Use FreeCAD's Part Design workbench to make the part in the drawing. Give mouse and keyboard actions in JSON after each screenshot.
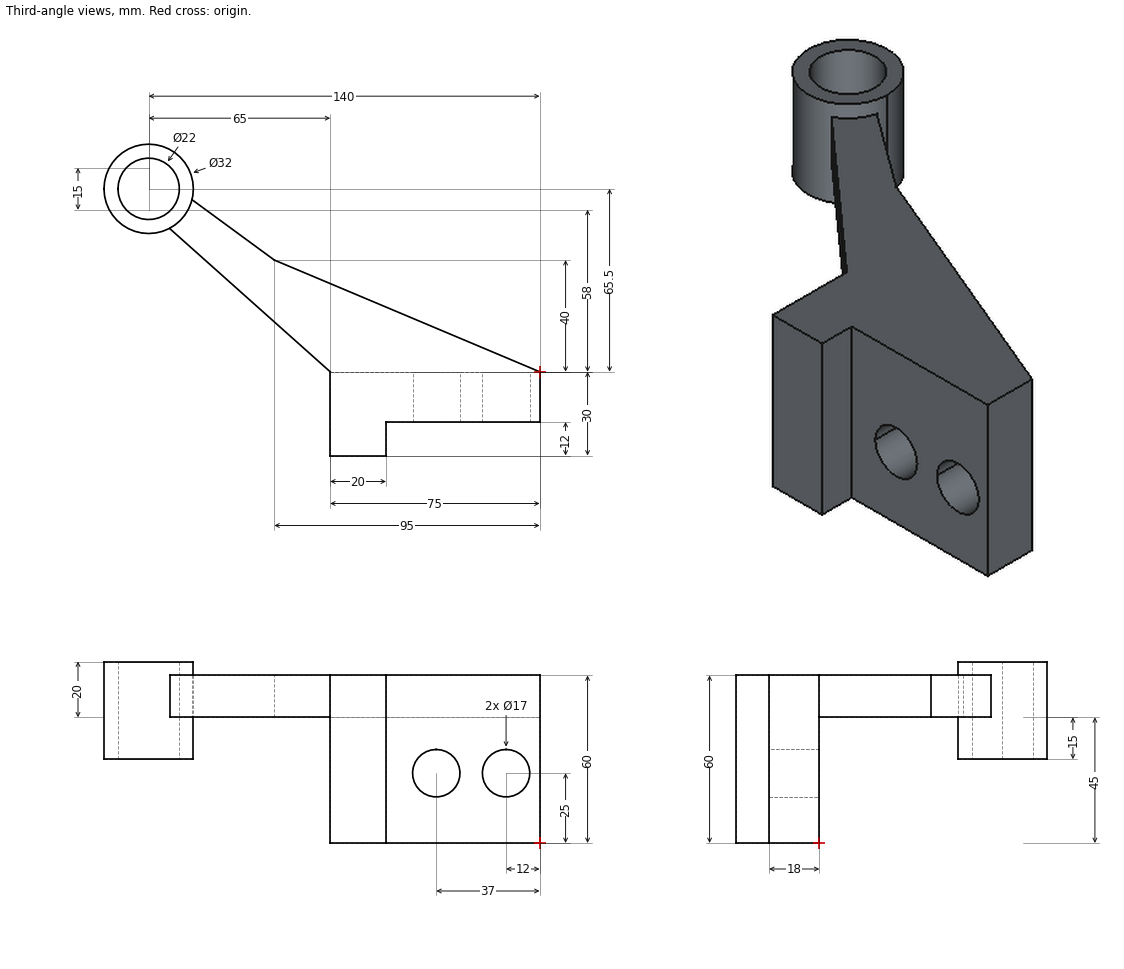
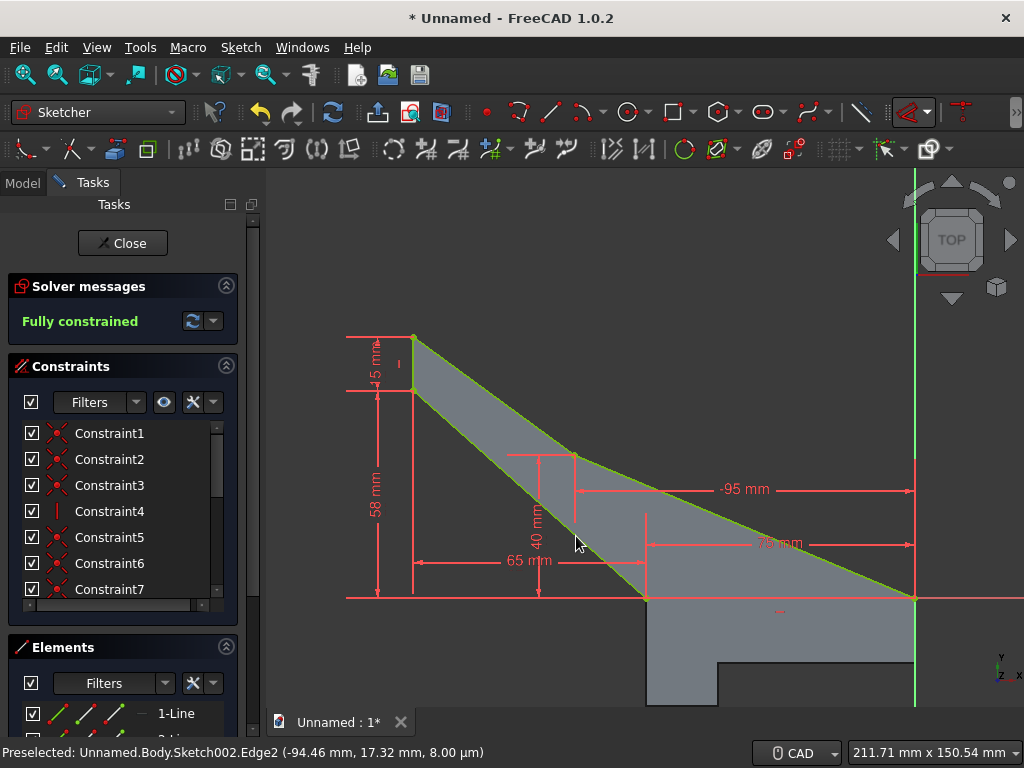
{"action": "left_click", "coordinate": [123, 243]}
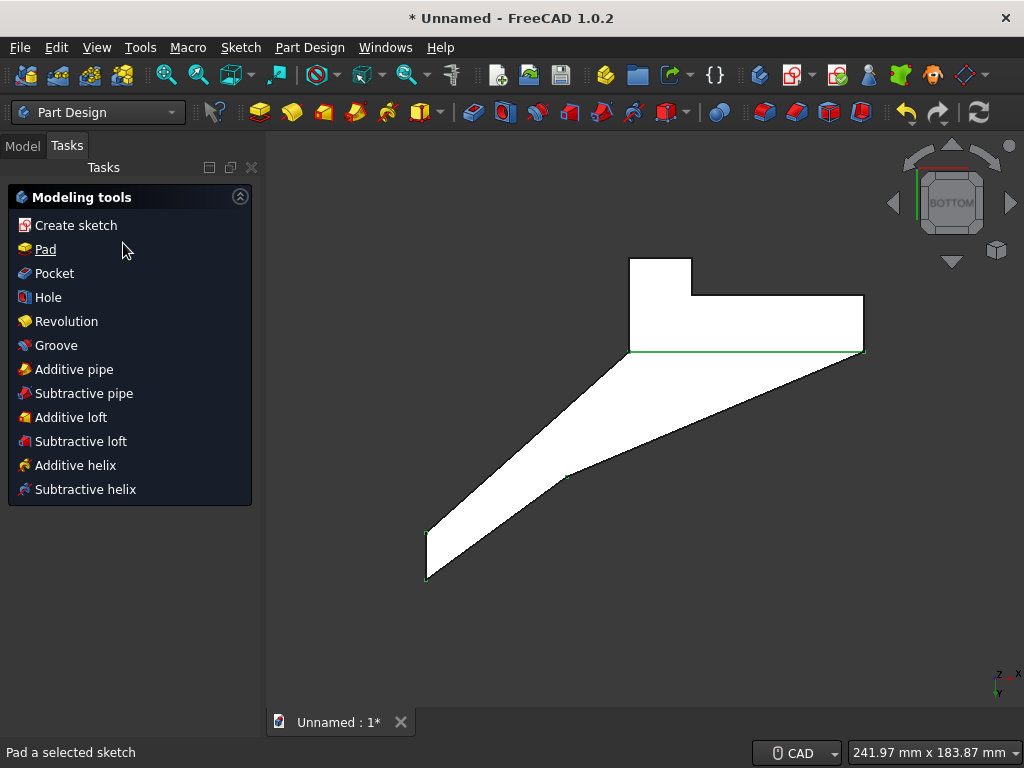
{"action": "left_click", "coordinate": [474, 112]}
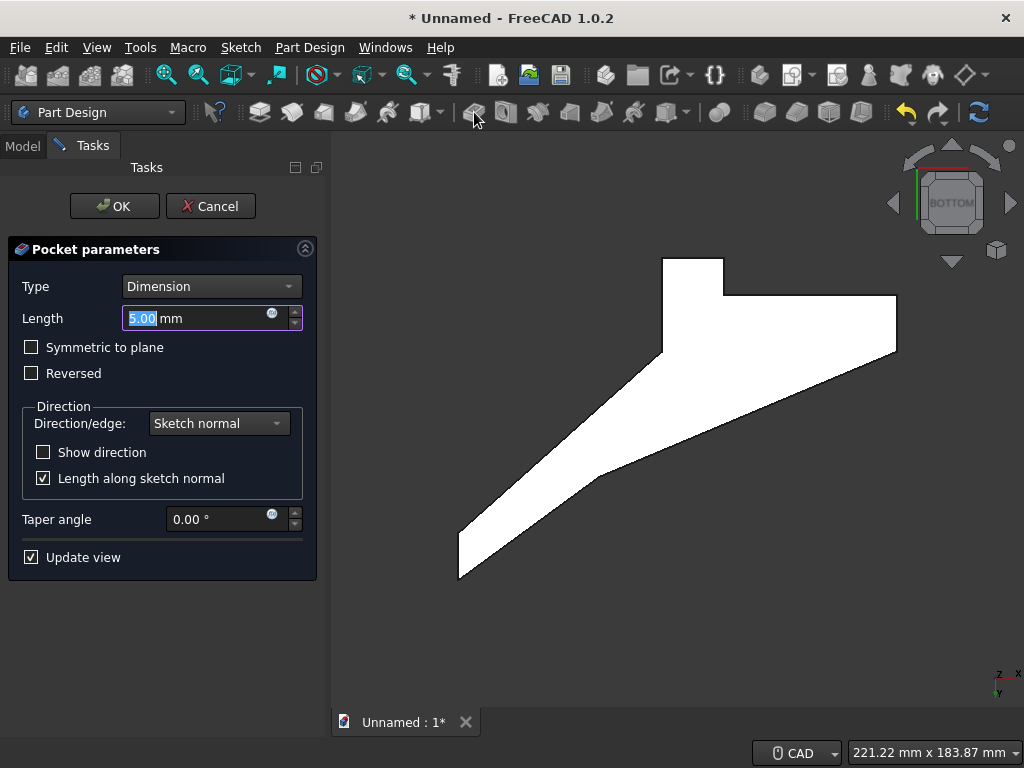
{"action": "type", "text": "45"}
{"action": "key", "text": "Tab"}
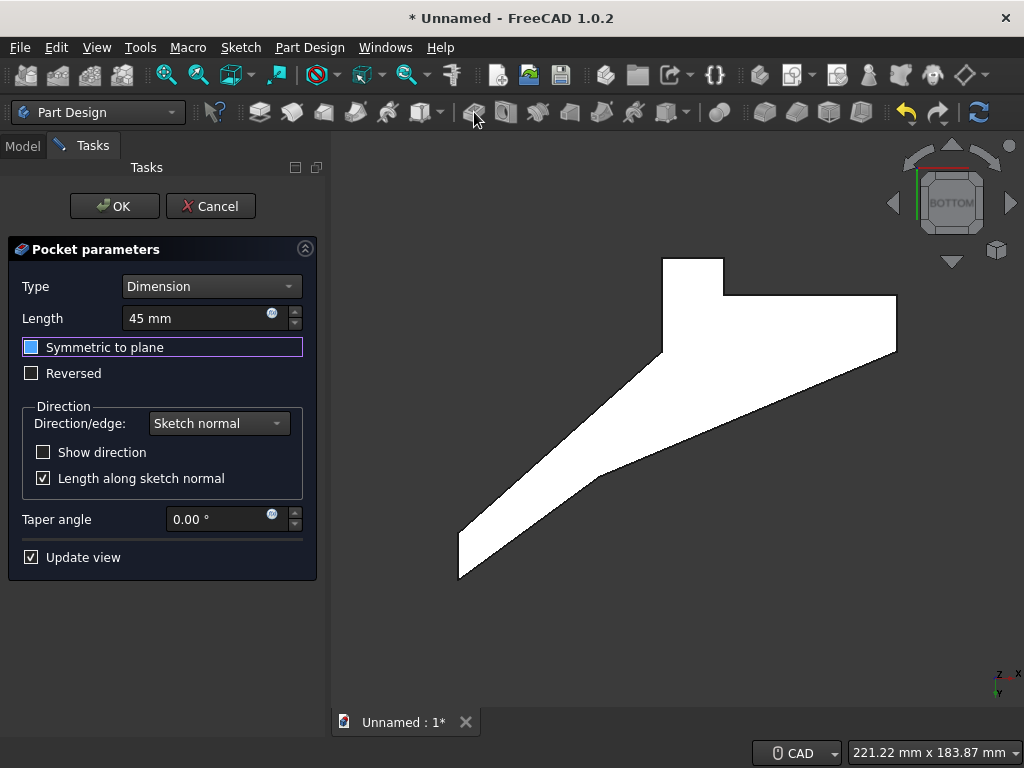
{"action": "left_click", "coordinate": [30, 373]}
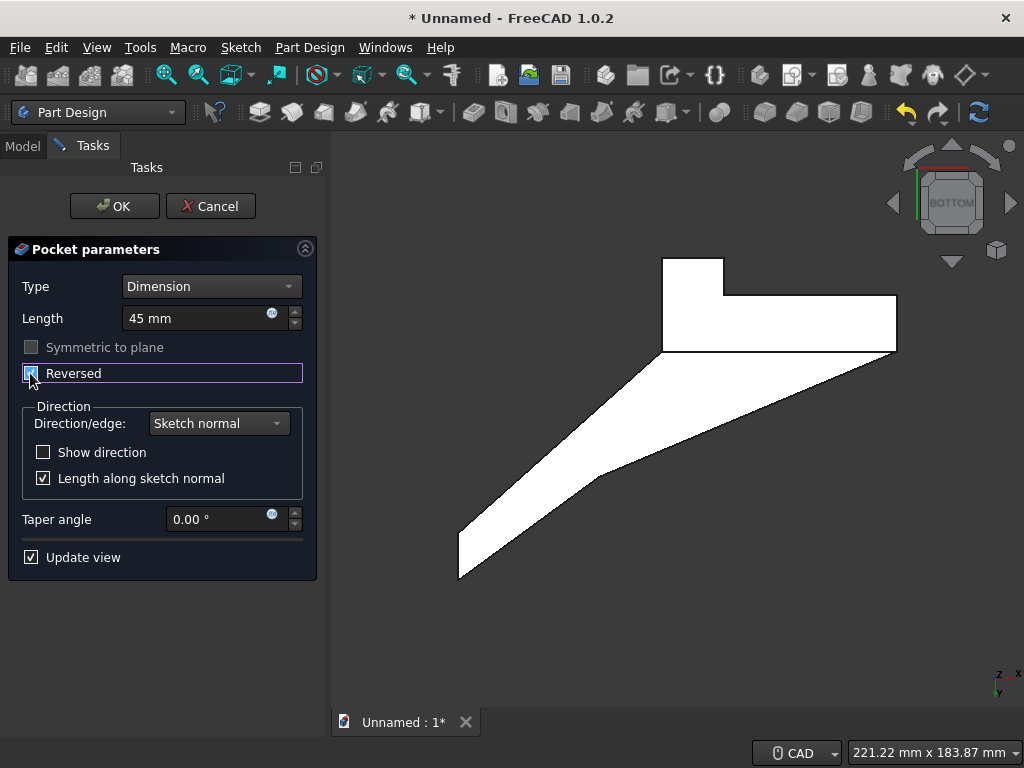
{"action": "left_click", "coordinate": [115, 206]}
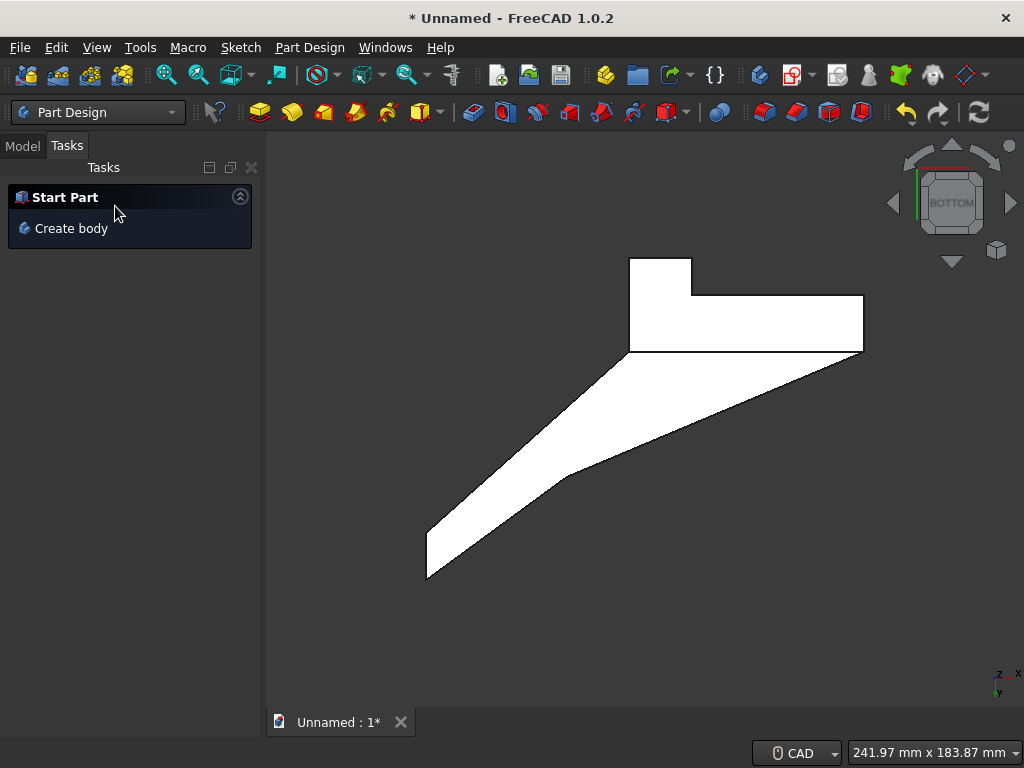
{"action": "left_click", "coordinate": [645, 400]}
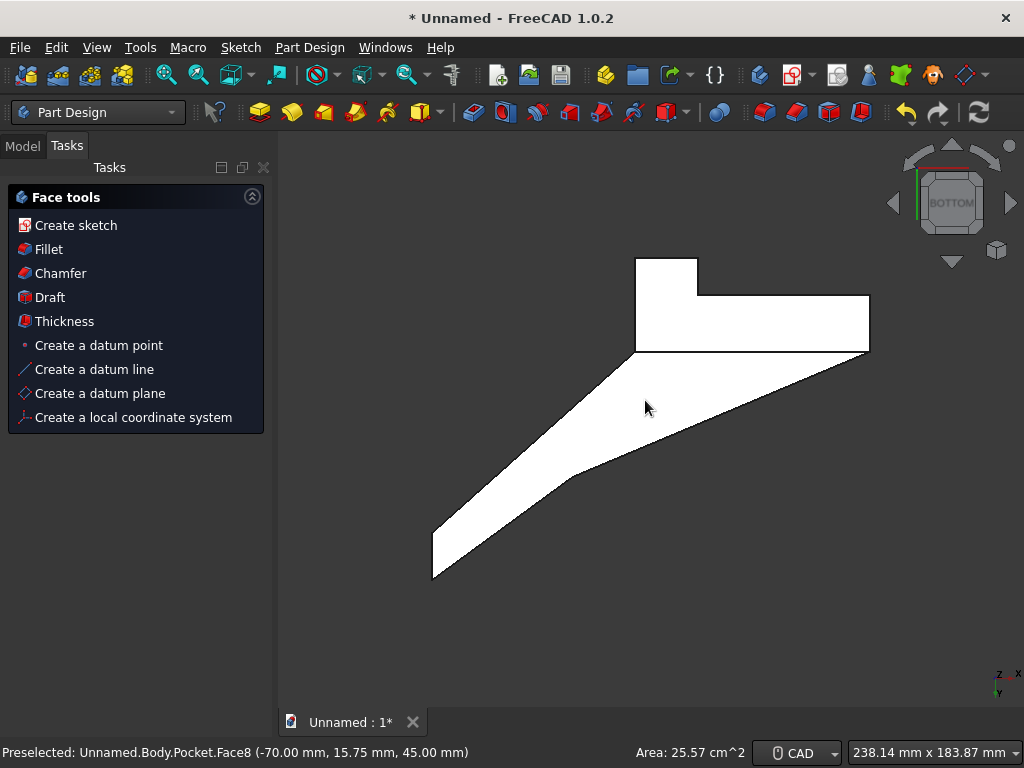
{"action": "left_click", "coordinate": [792, 76]}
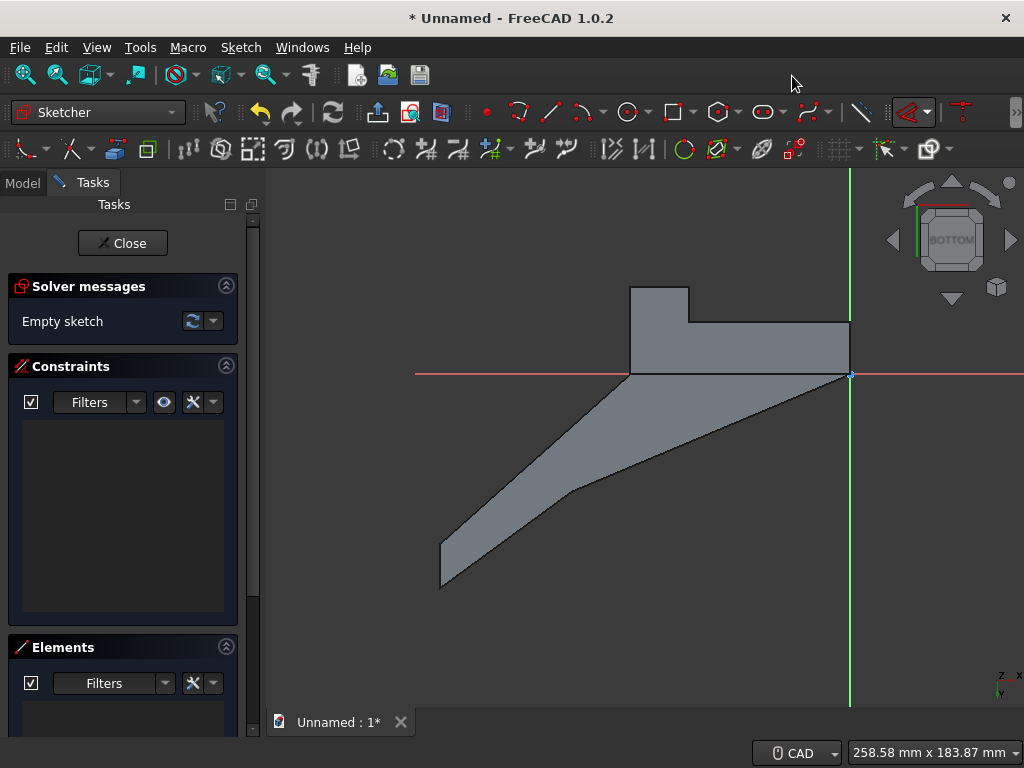
{"action": "scroll", "coordinate": [381, 622], "scroll_direction": "up", "scroll_amount": 6}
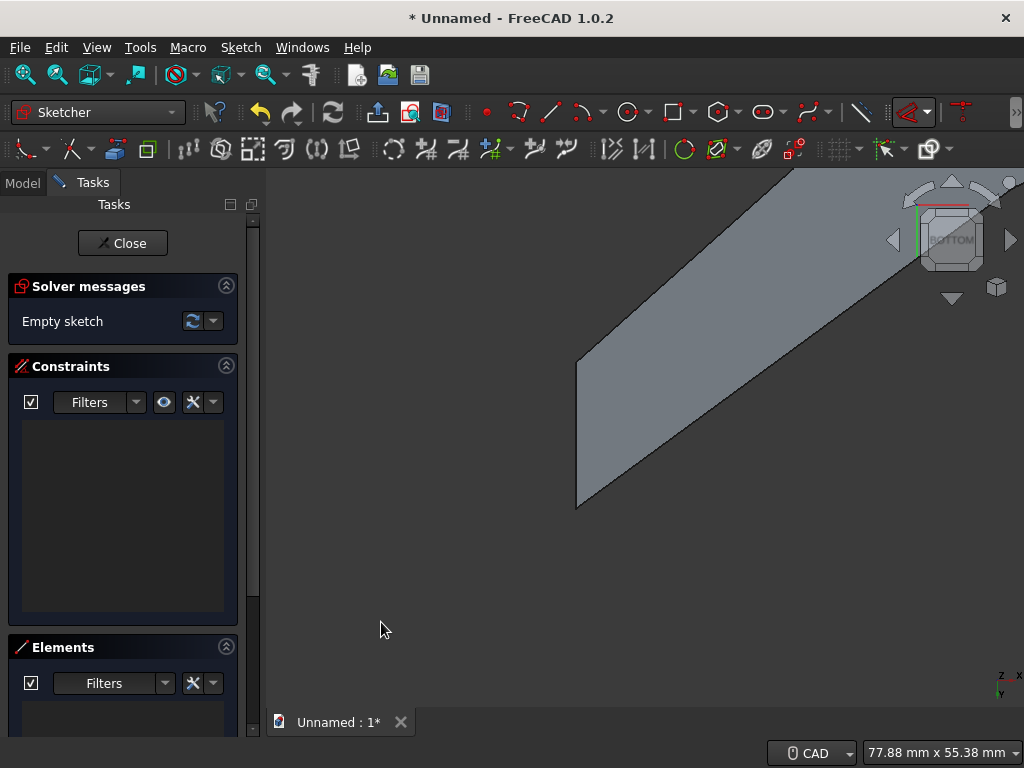
{"action": "left_click", "coordinate": [628, 112]}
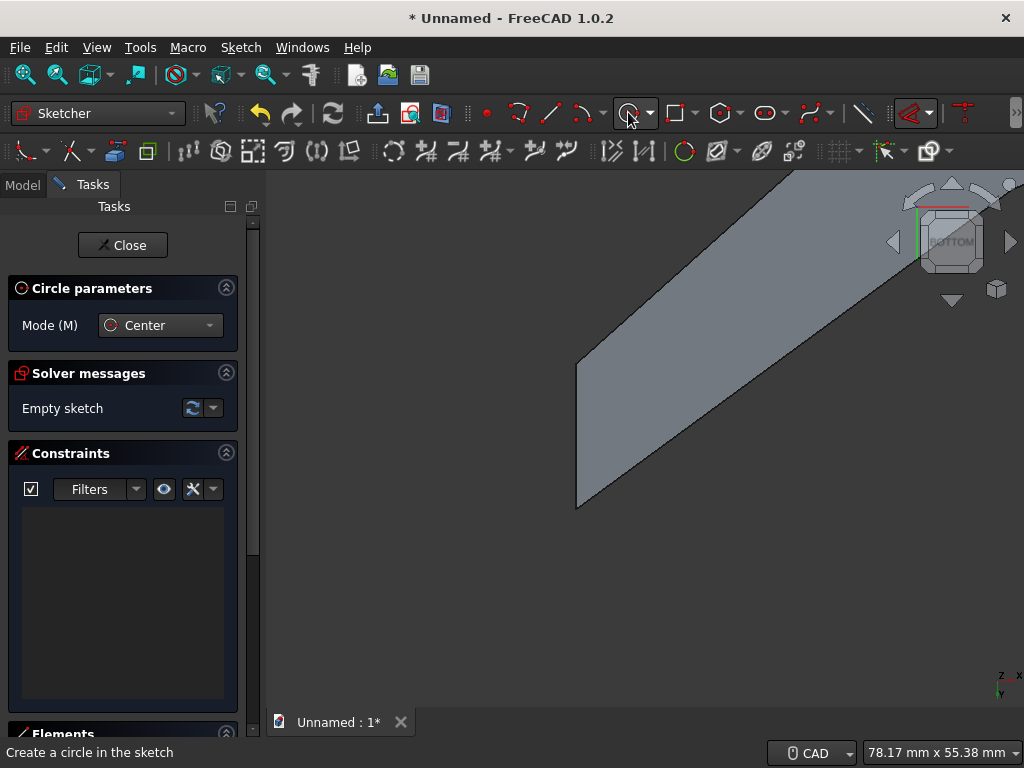
{"action": "left_click", "coordinate": [576, 437]}
{"action": "left_click", "coordinate": [686, 327]}
{"action": "key", "text": "Escape"}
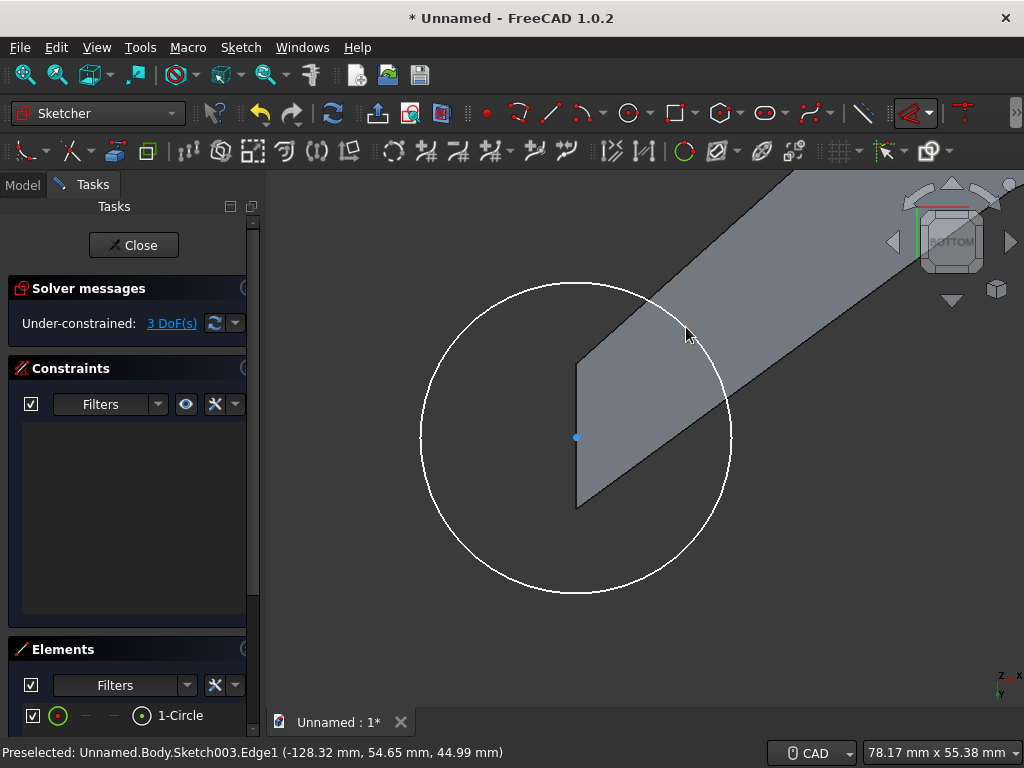
{"action": "left_click", "coordinate": [686, 328]}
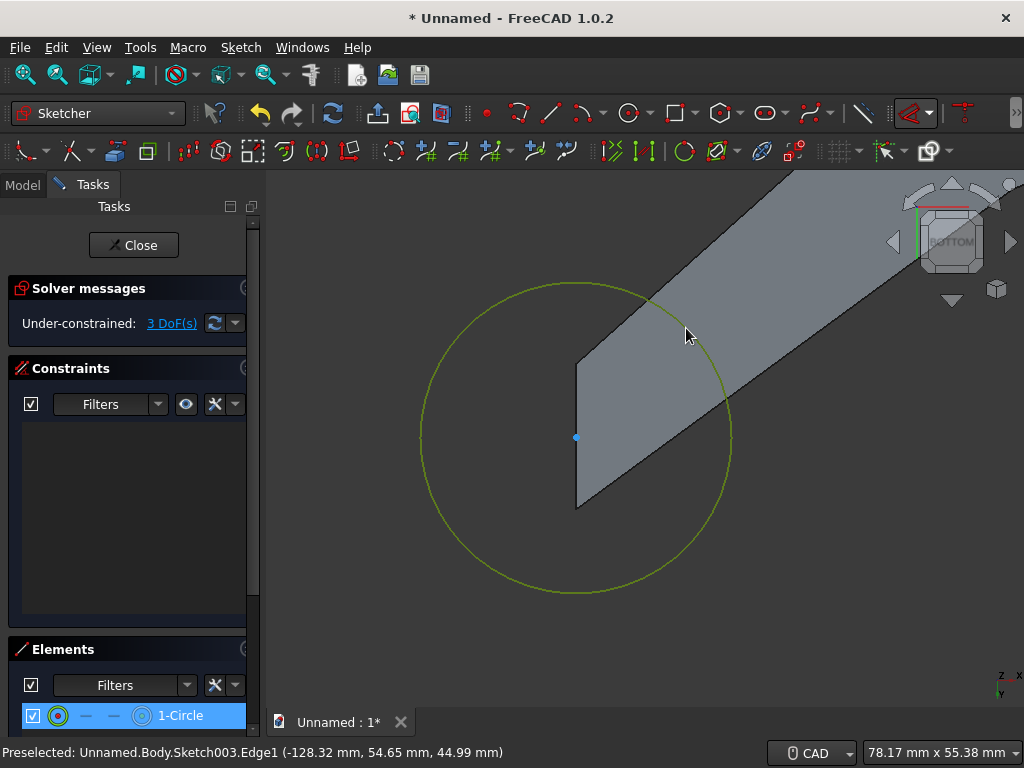
{"action": "key", "text": "k o"}